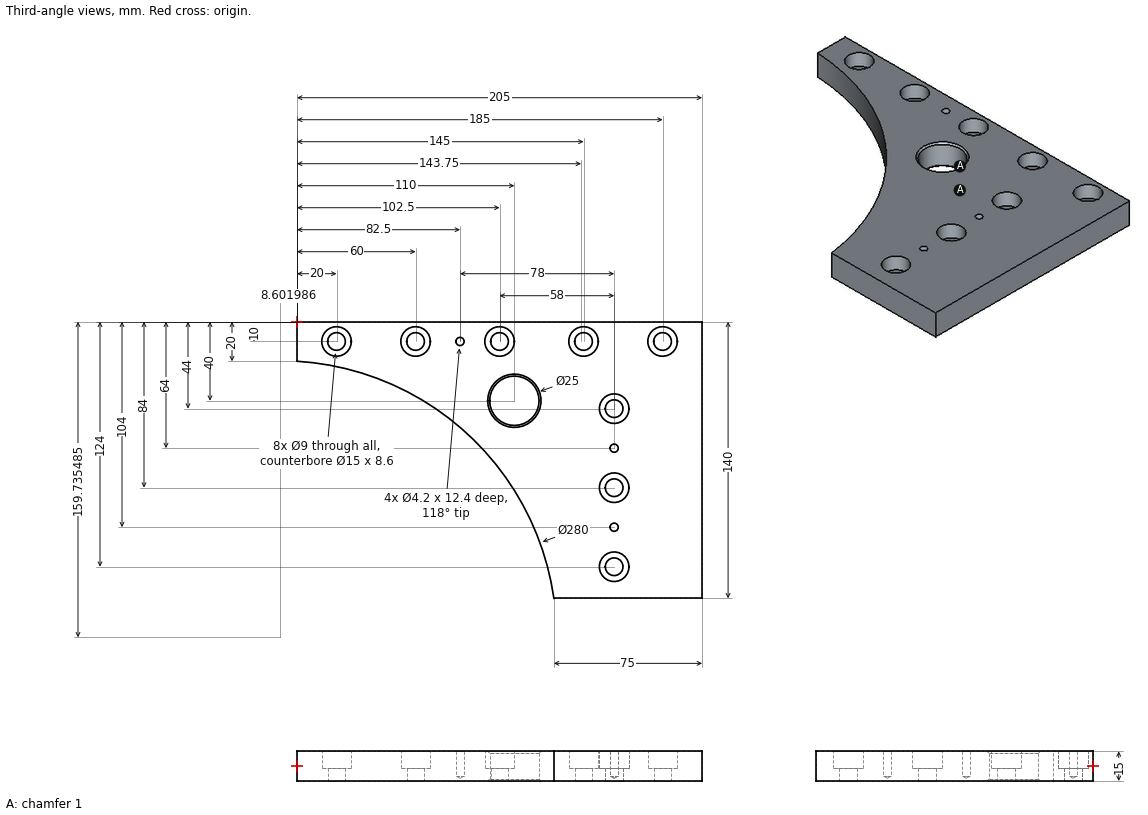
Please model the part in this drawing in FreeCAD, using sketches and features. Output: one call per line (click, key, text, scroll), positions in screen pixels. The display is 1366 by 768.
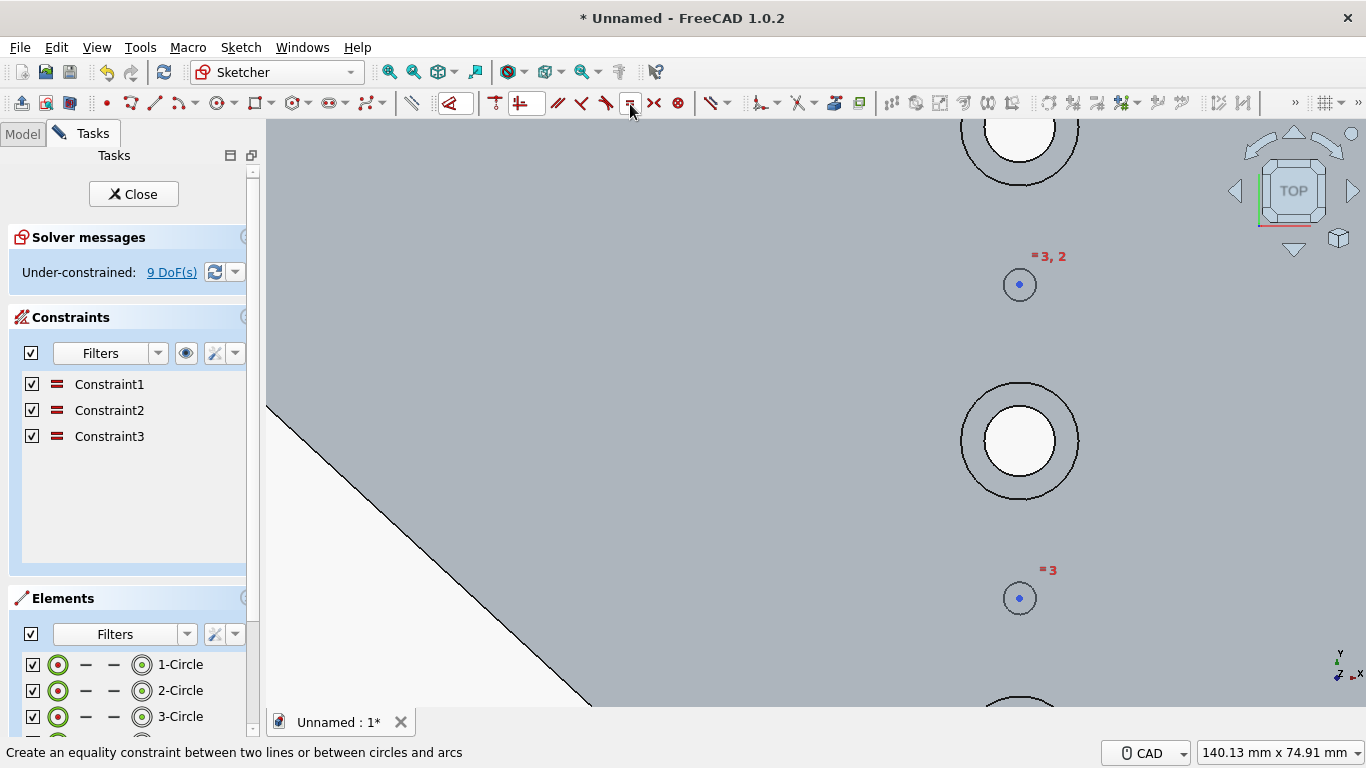
scroll(1033, 588, down, 4)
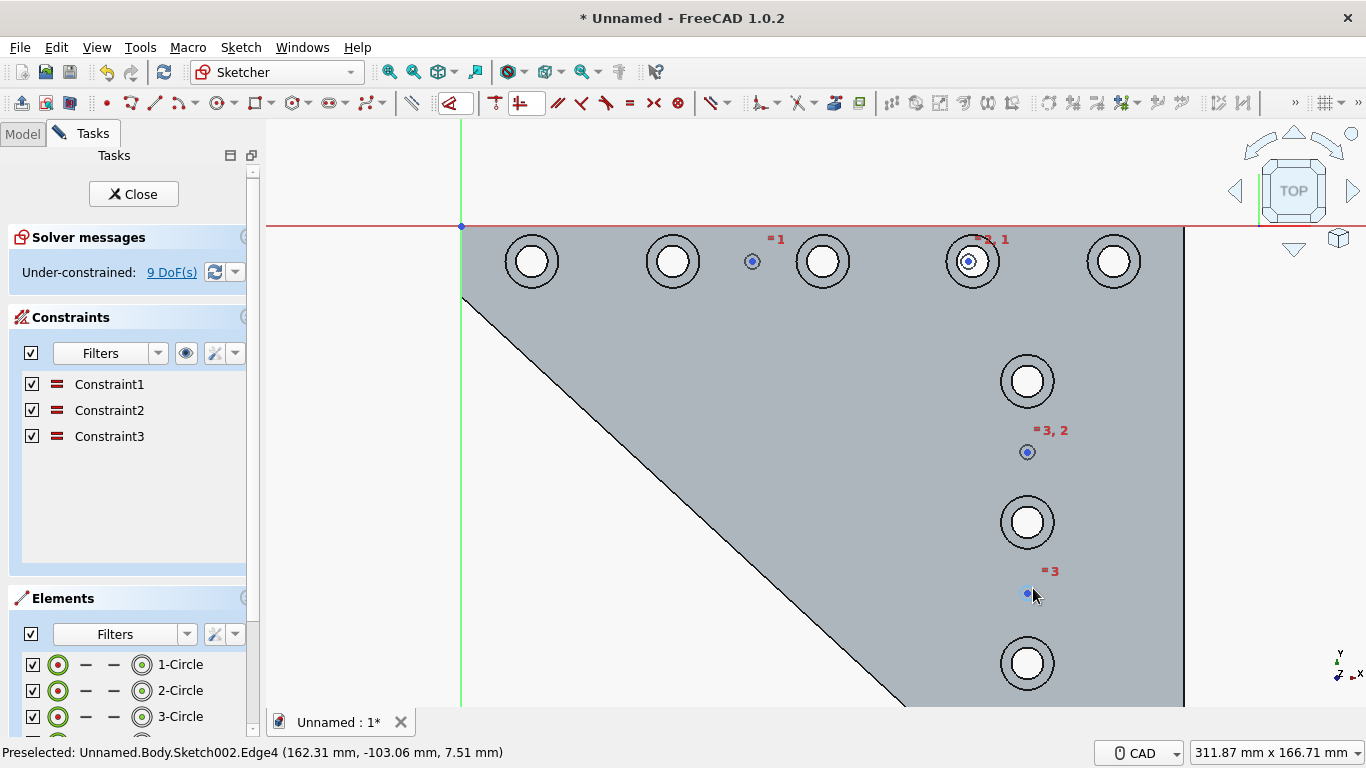
click(752, 262)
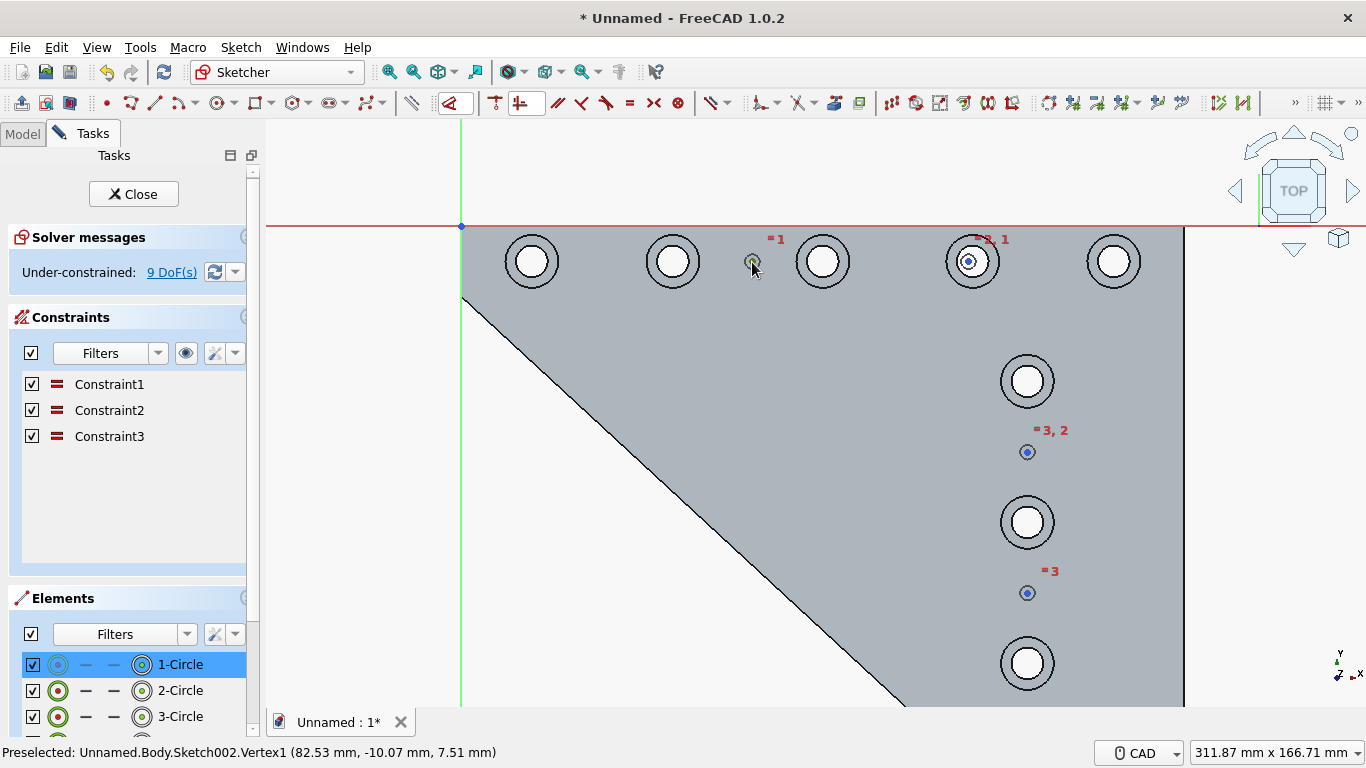
click(968, 262)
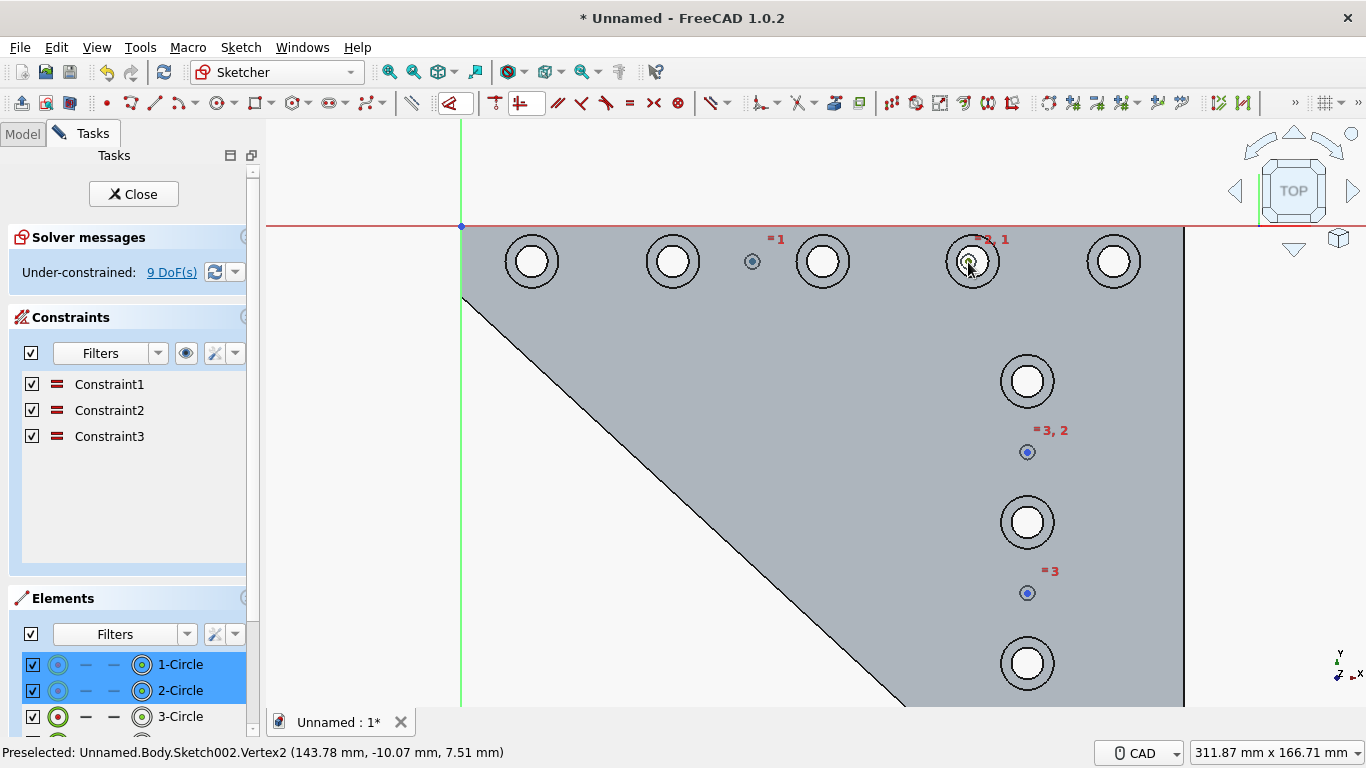
click(540, 104)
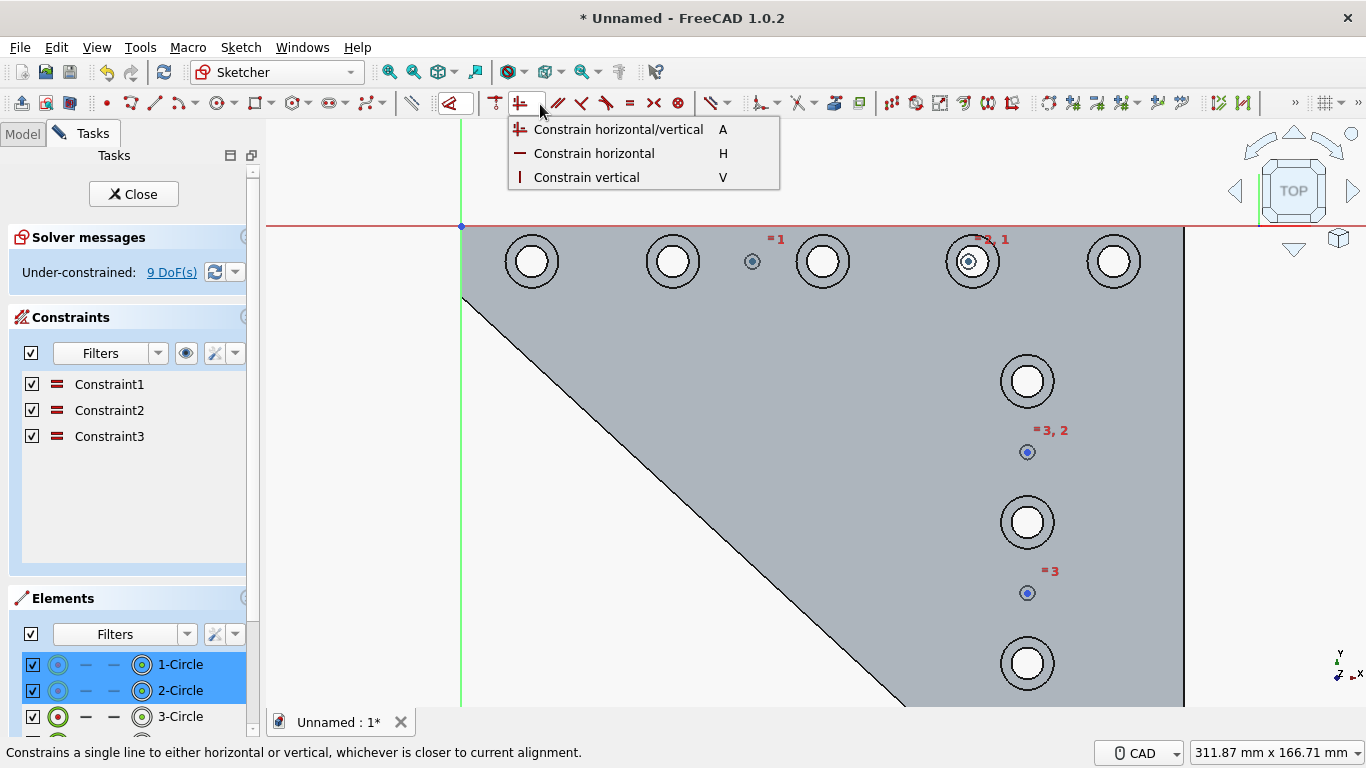
click(644, 153)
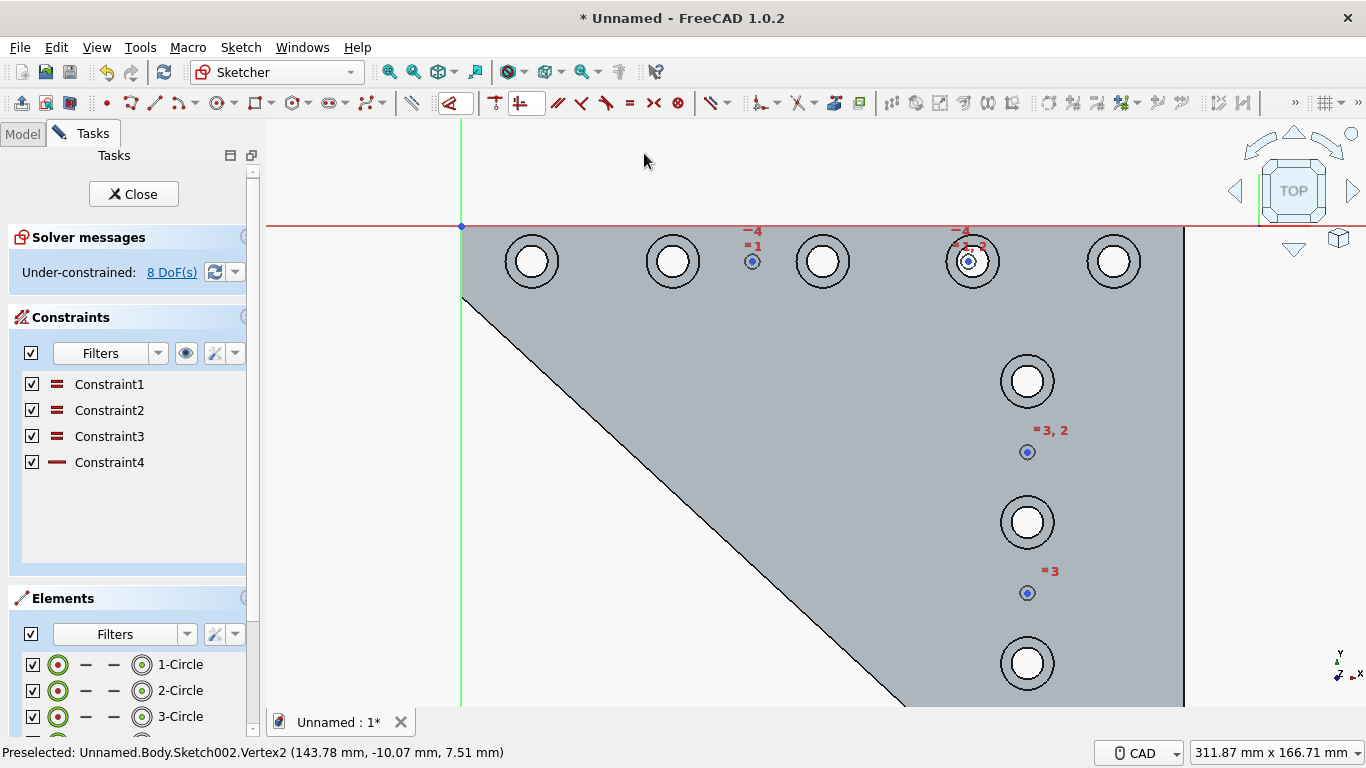
click(1027, 452)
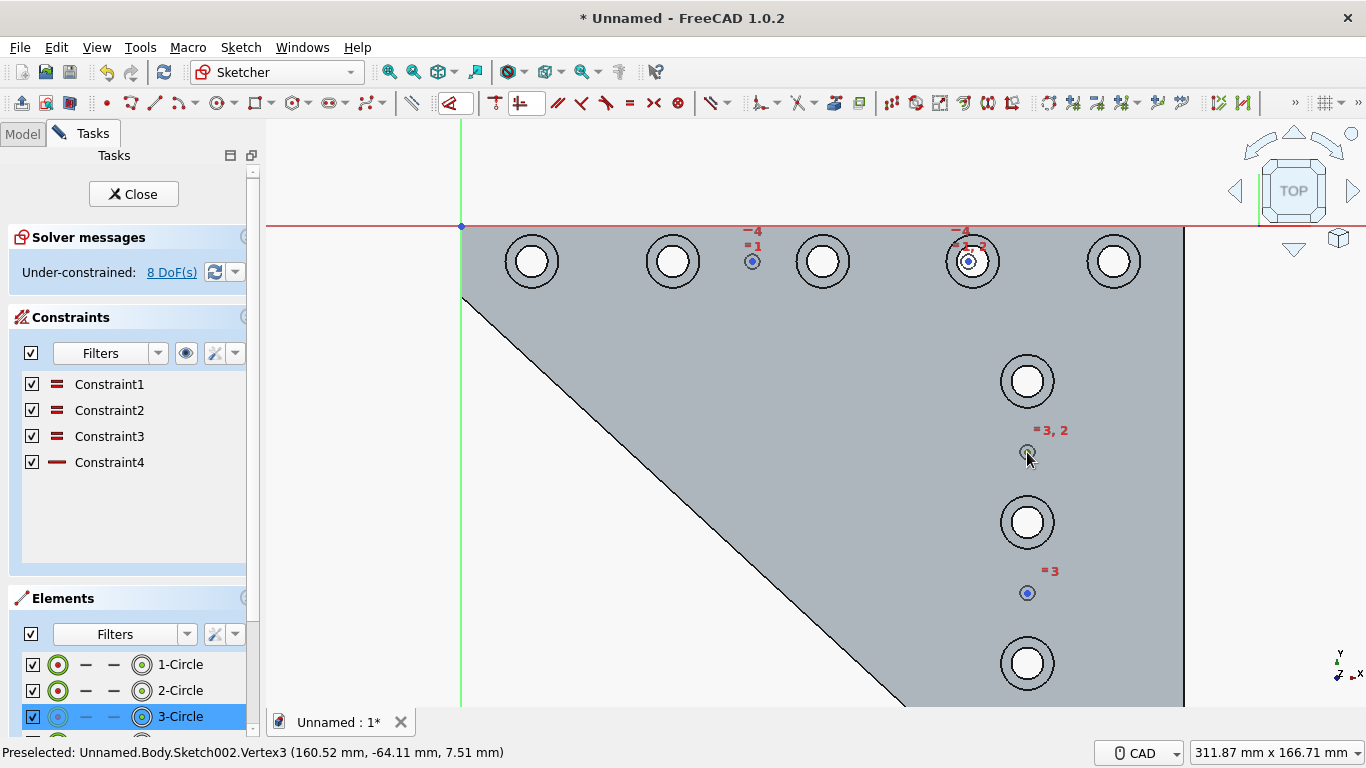
click(1027, 593)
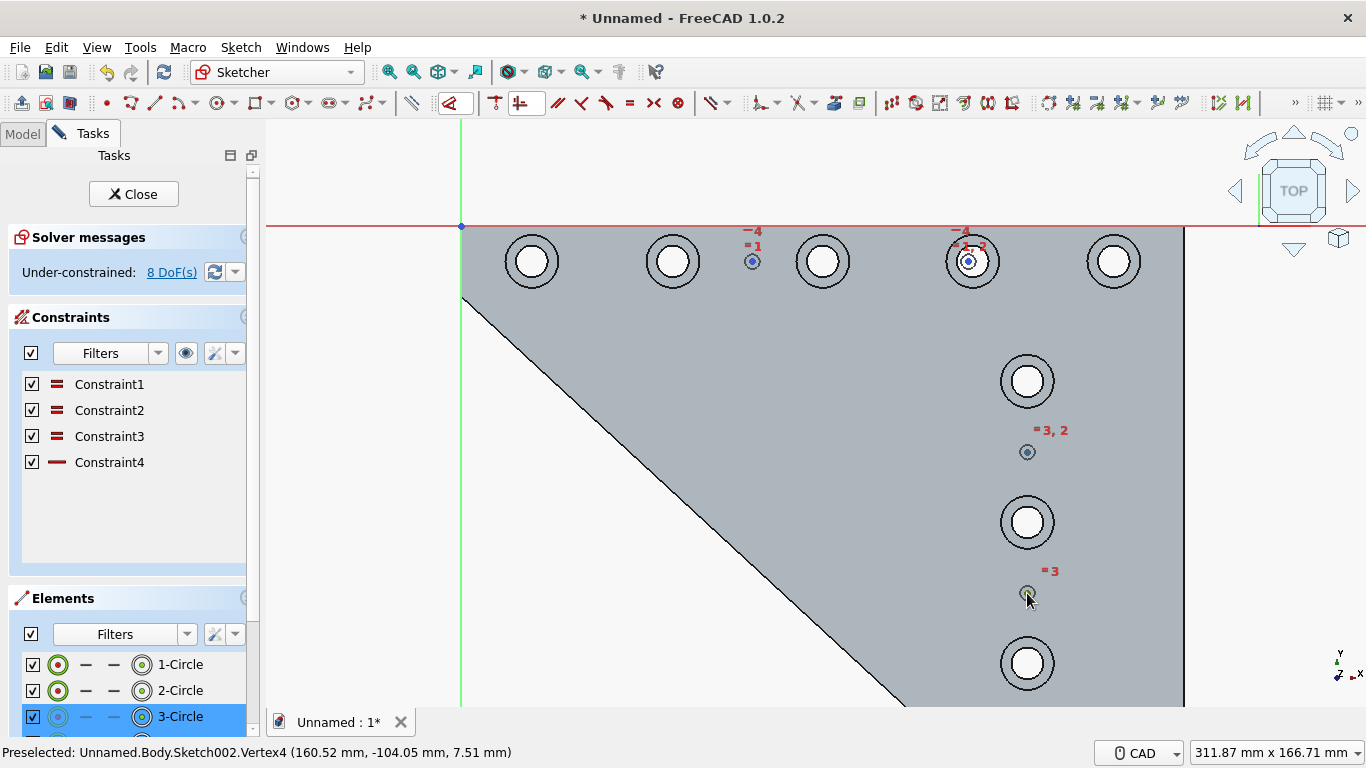
click(540, 104)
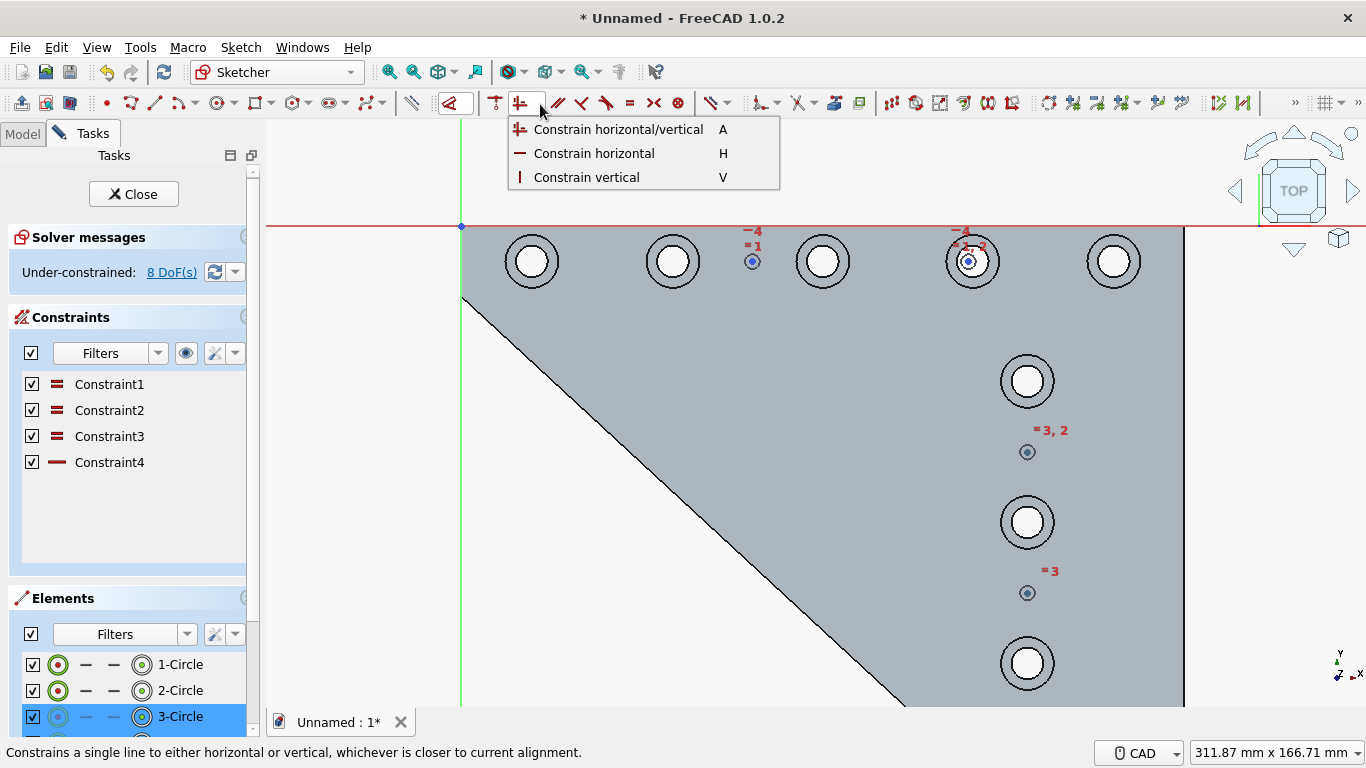
click(644, 177)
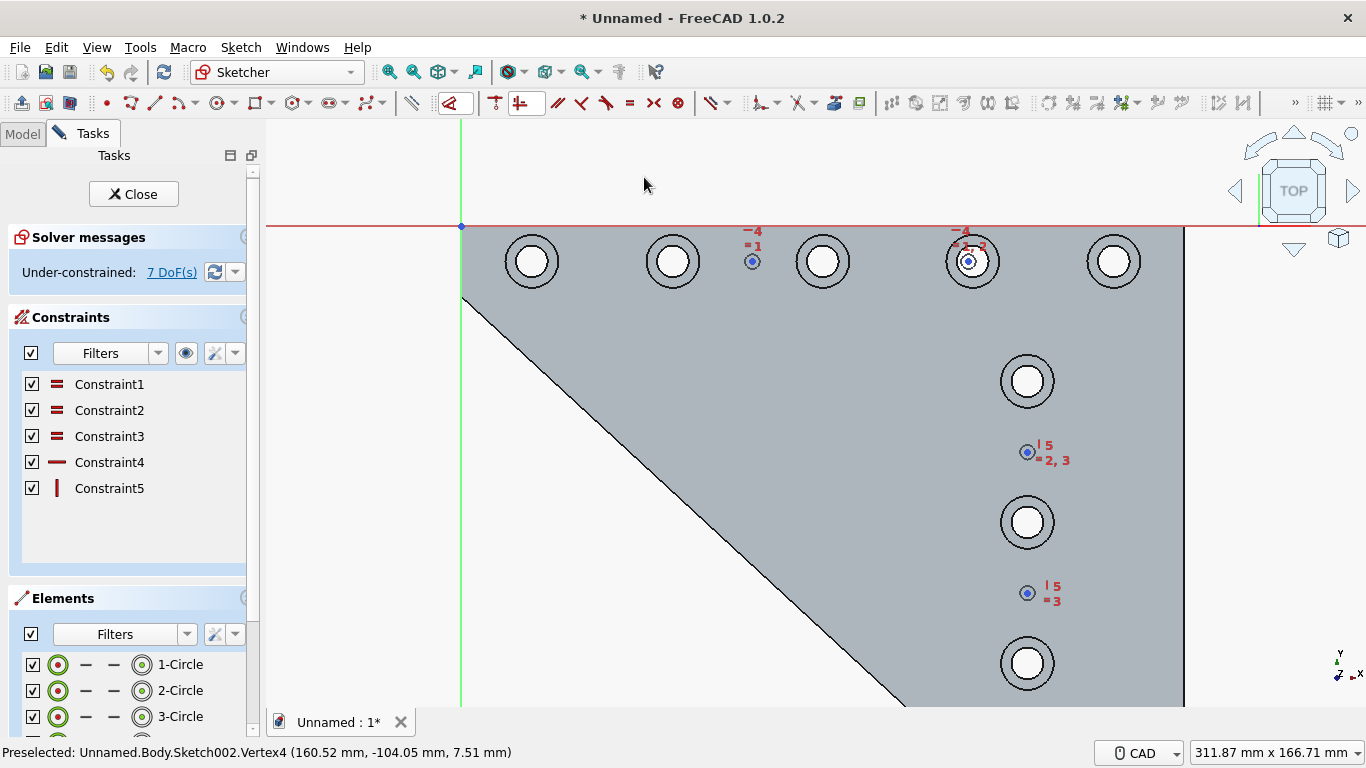
scroll(747, 257, up, 5)